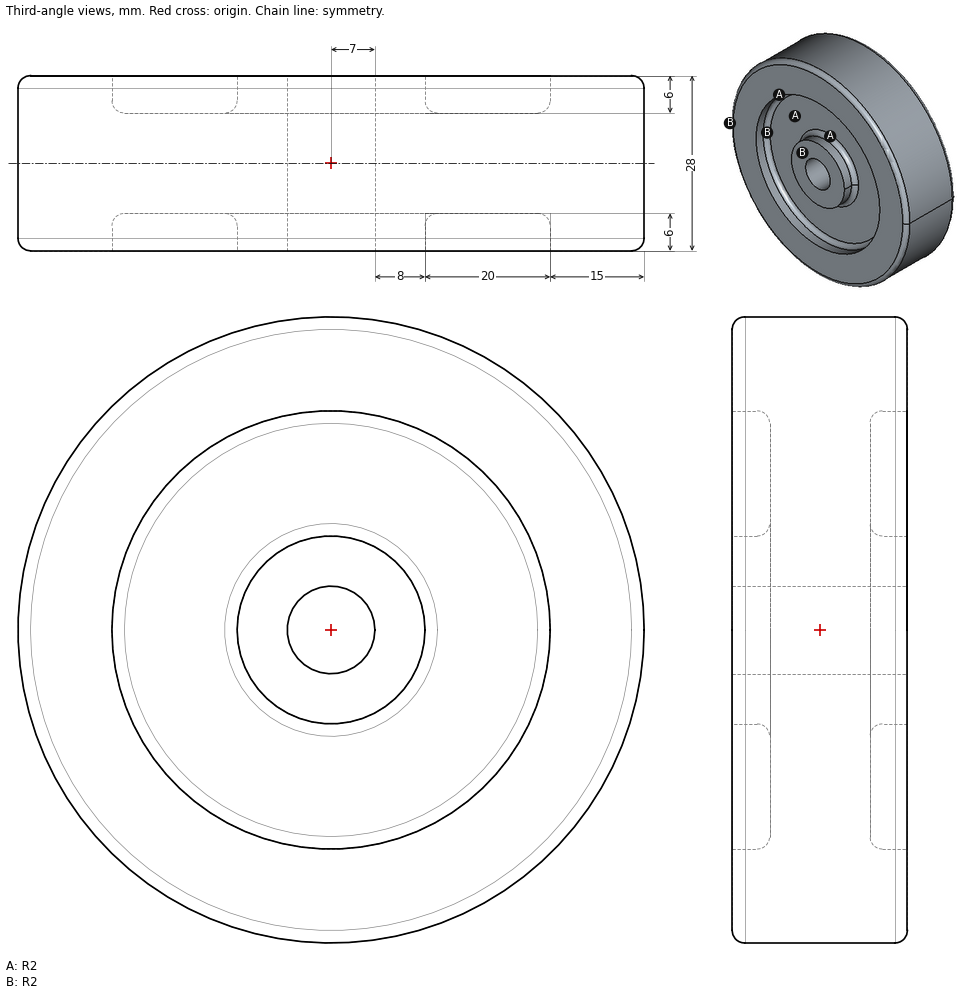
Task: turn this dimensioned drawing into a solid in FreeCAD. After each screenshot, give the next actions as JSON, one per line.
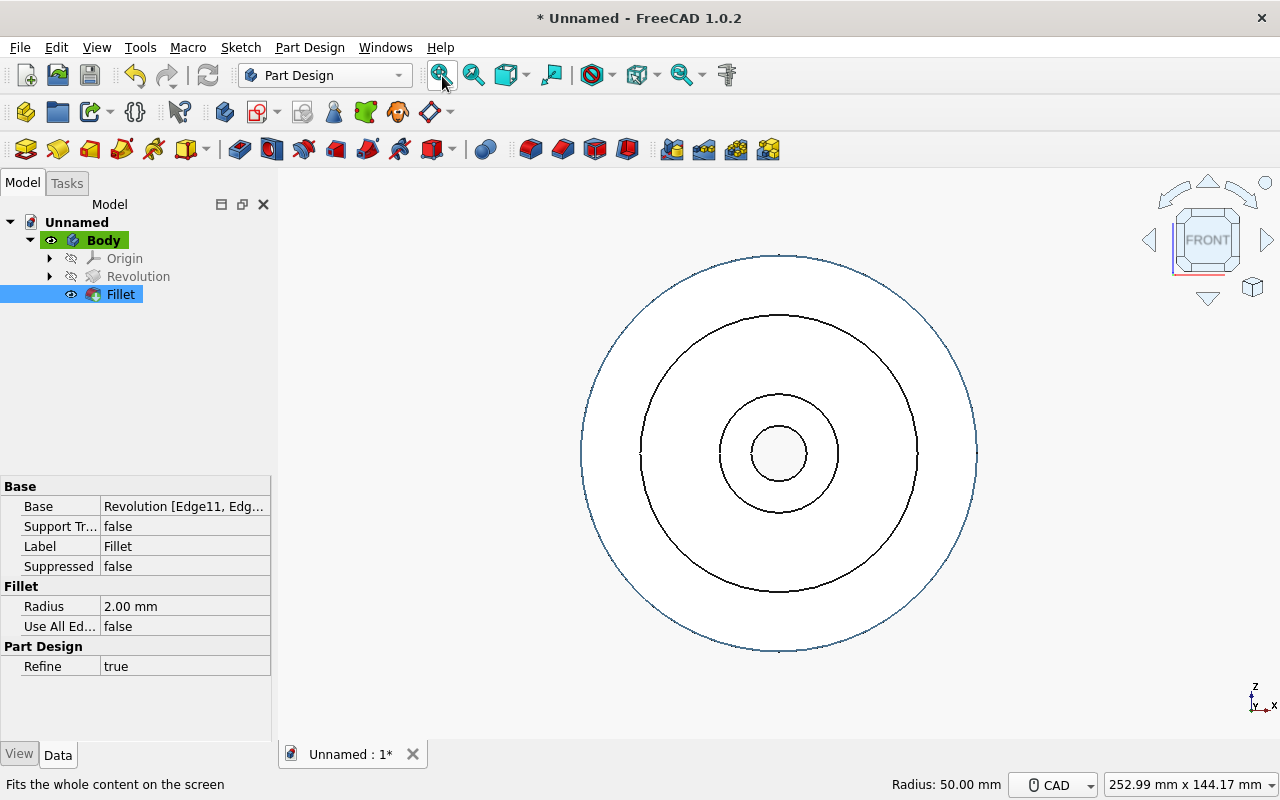
{"action": "key", "text": "3"}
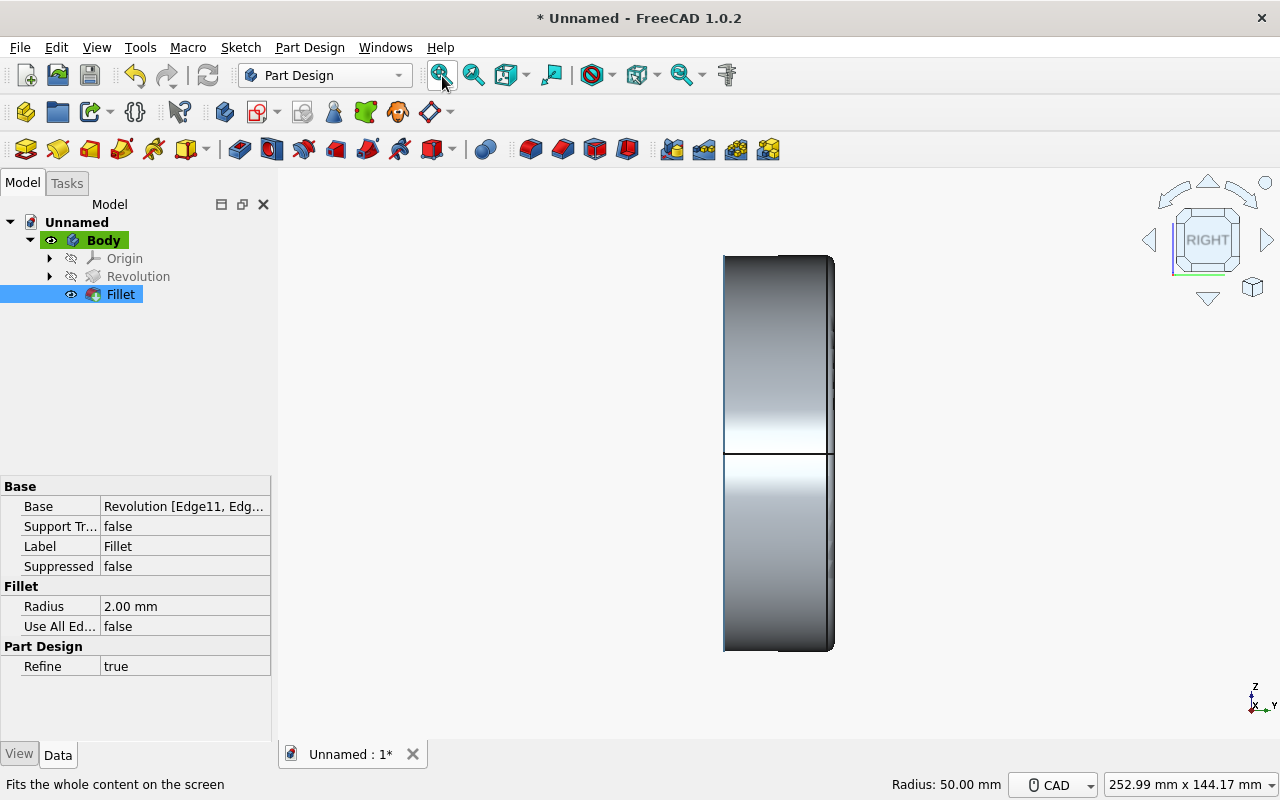
{"action": "key", "text": "5"}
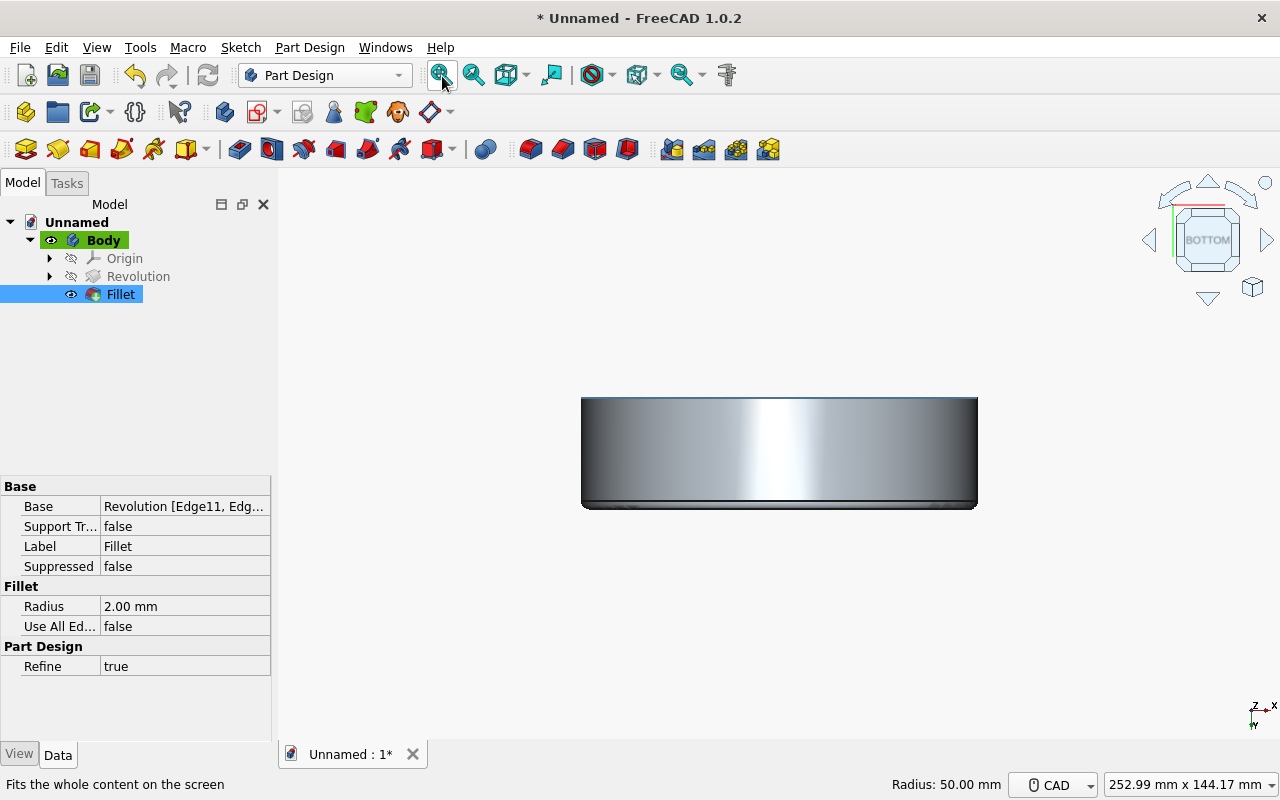
{"action": "left_click", "coordinate": [442, 76]}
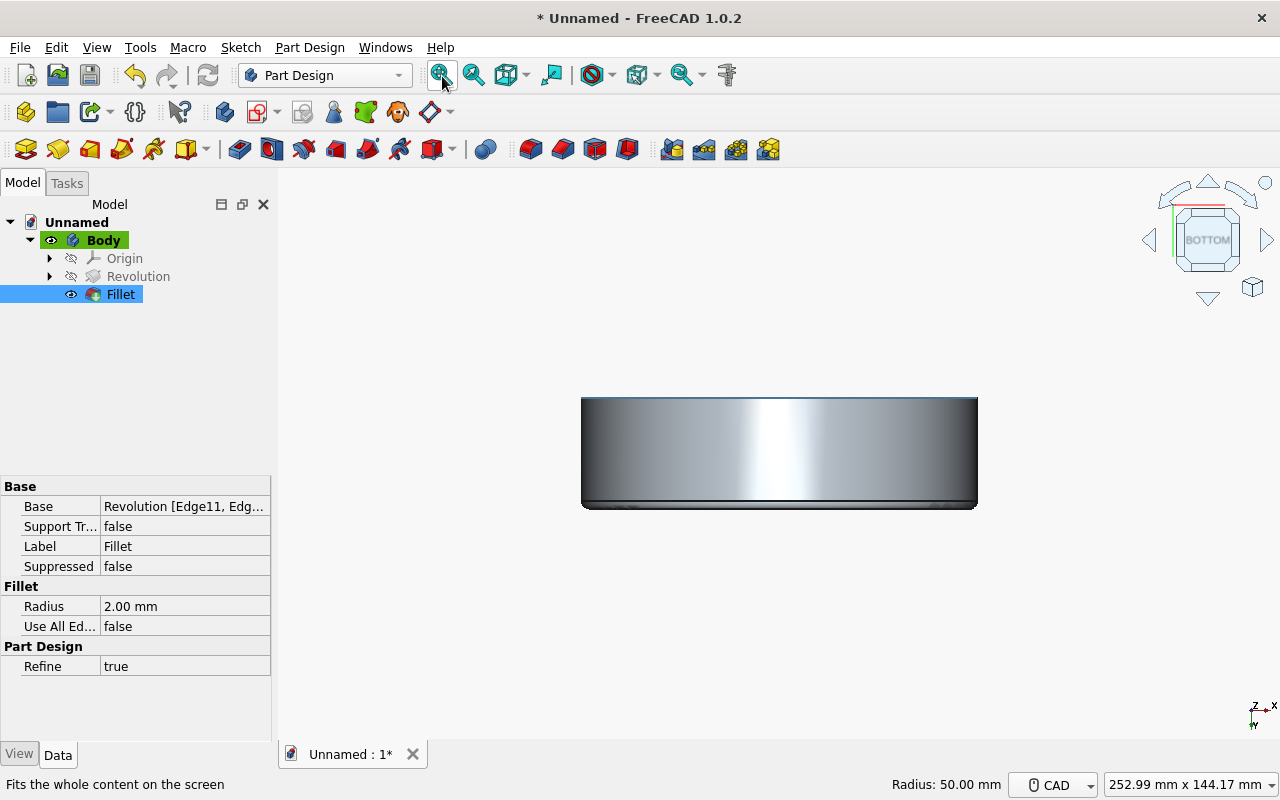
{"action": "key", "text": "4"}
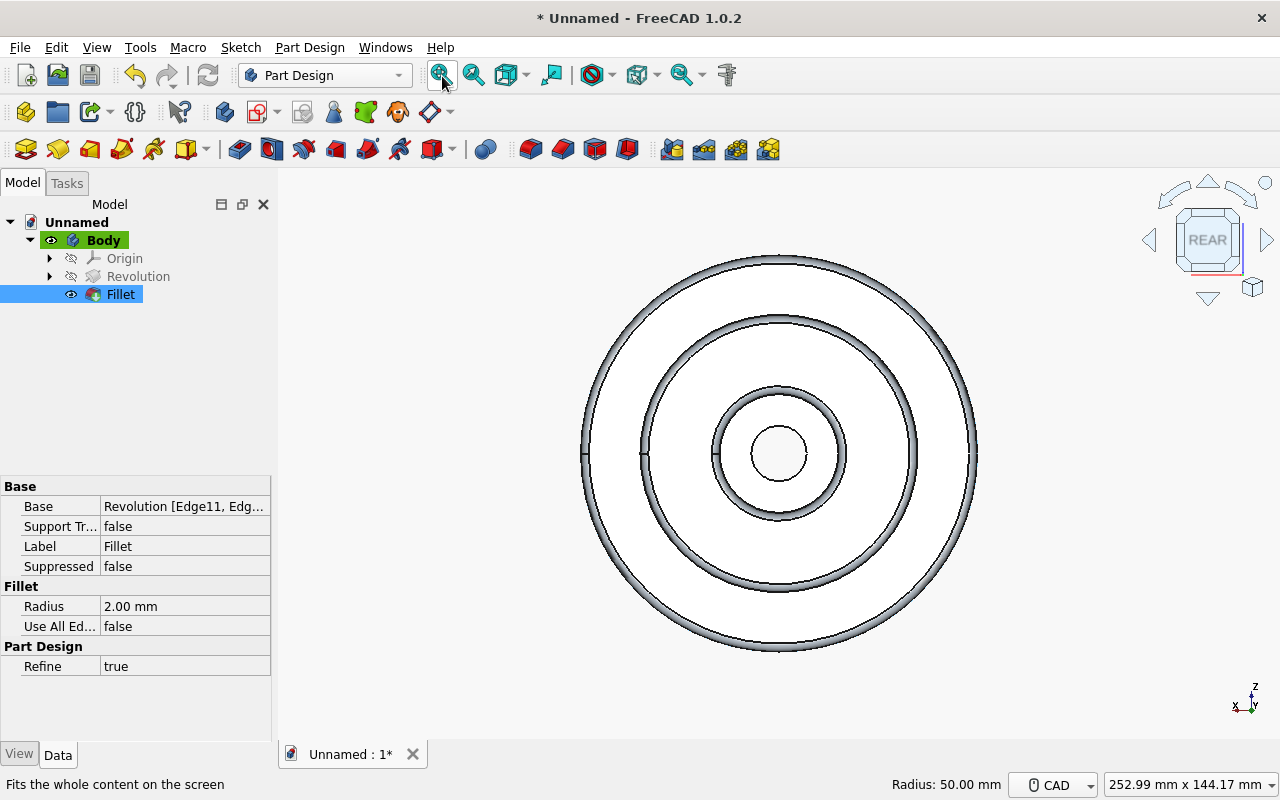
{"action": "key", "text": "6"}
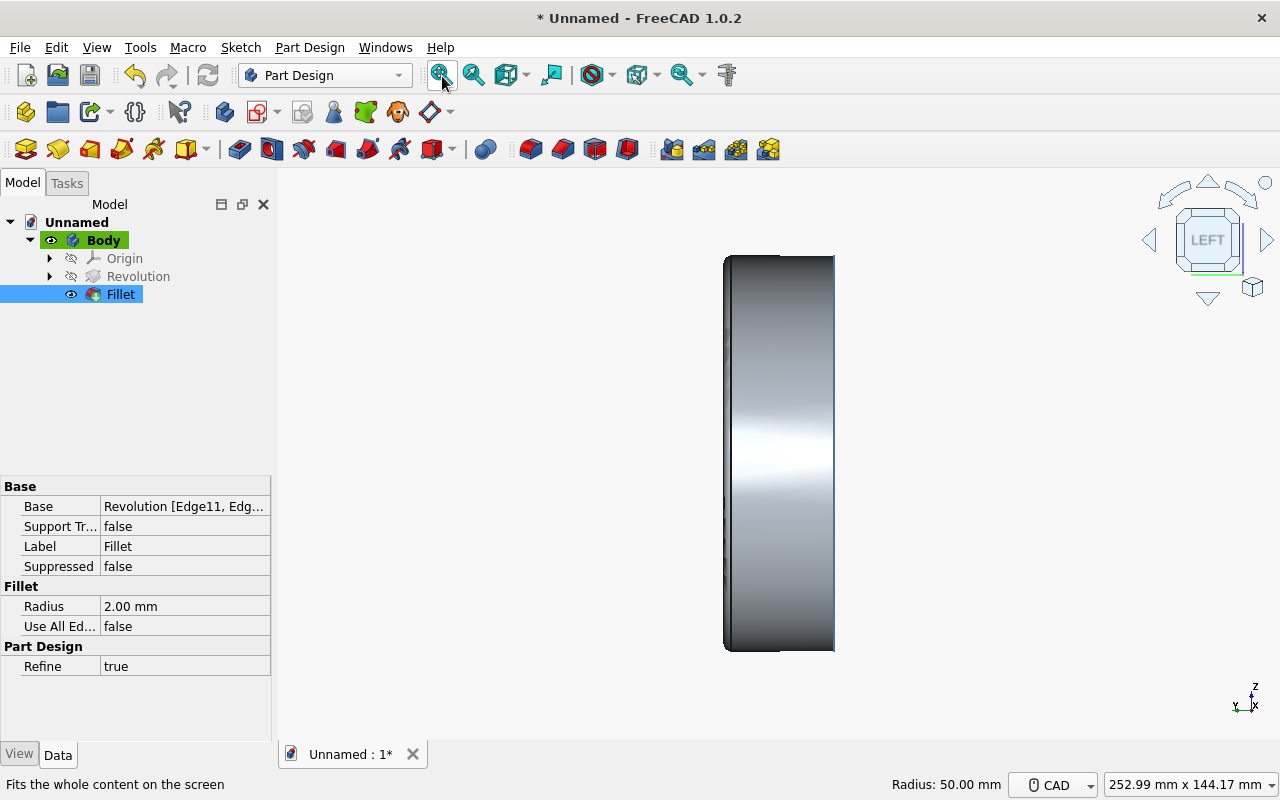
{"action": "key", "text": "v 3"}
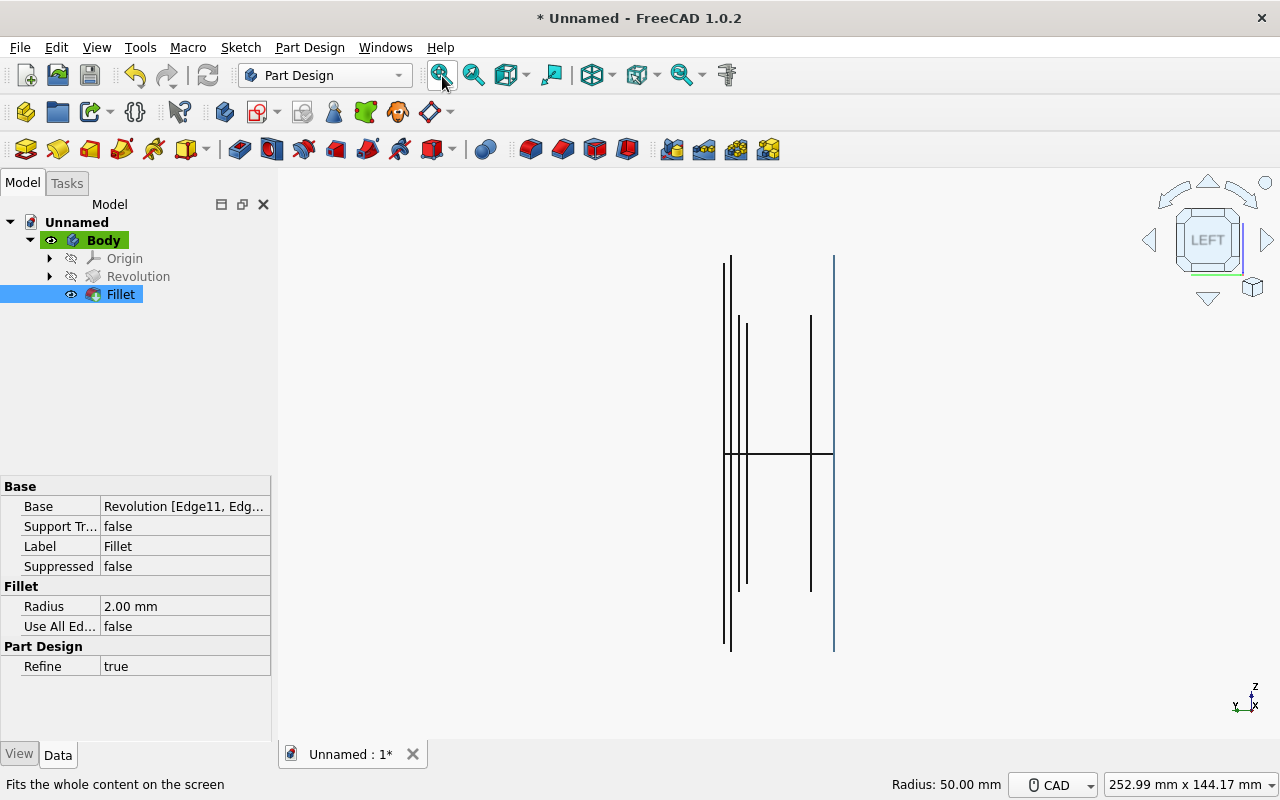
{"action": "key", "text": "0"}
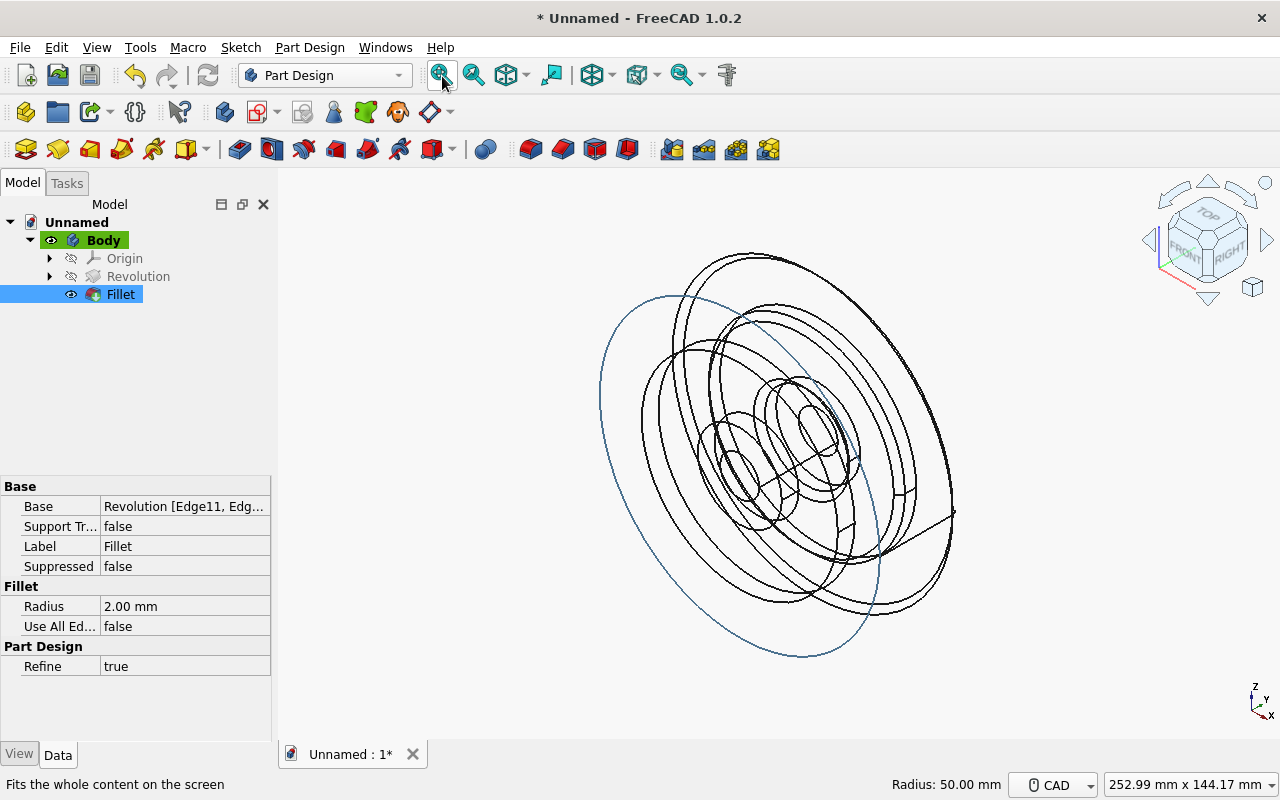
{"action": "left_click", "coordinate": [659, 409], "text": "ctrl"}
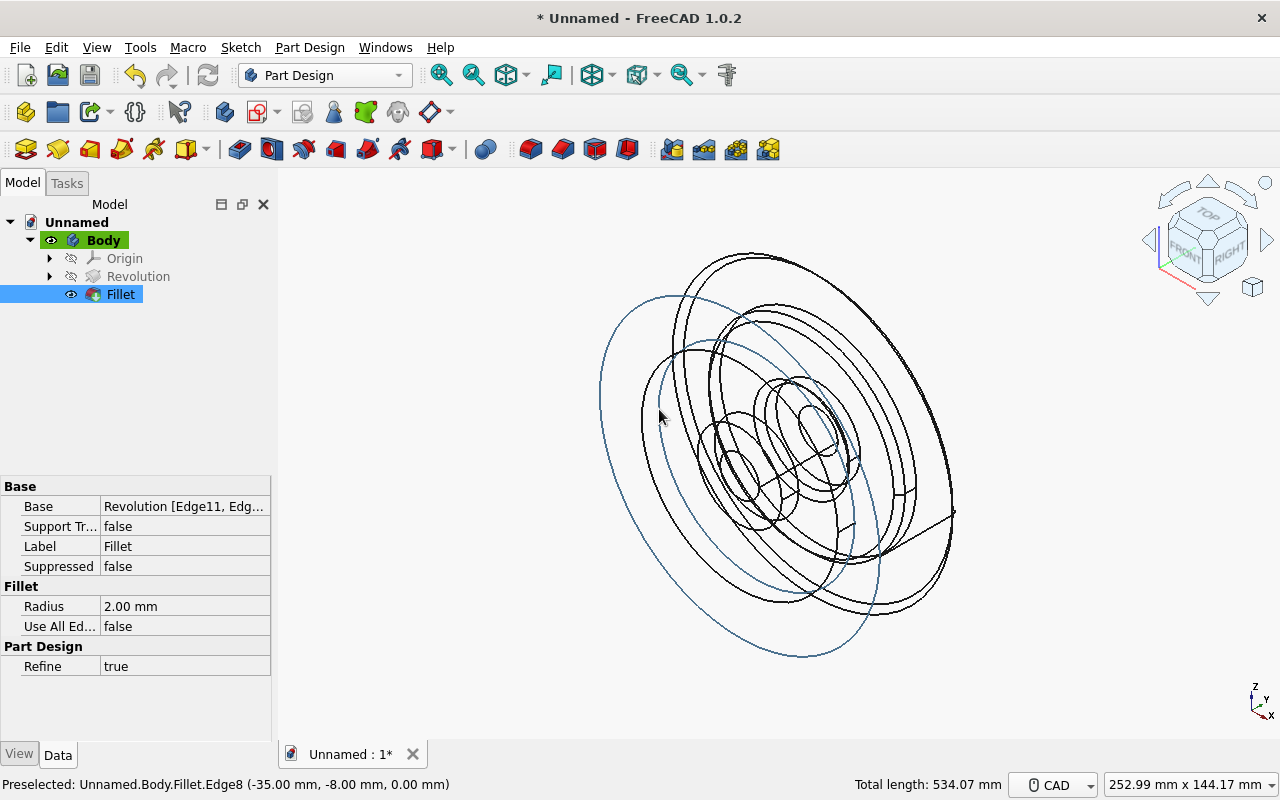
{"action": "left_click", "coordinate": [715, 441], "text": "ctrl"}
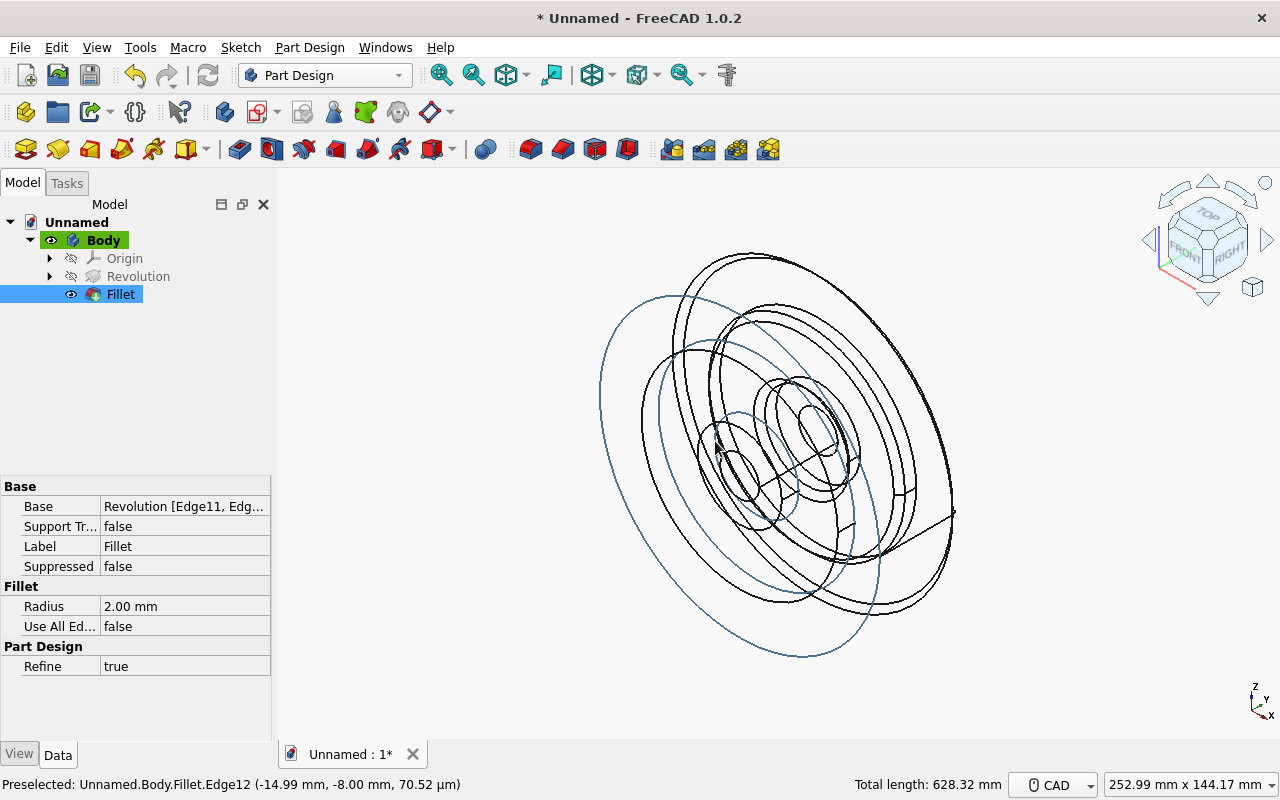
{"action": "key", "text": "v 1"}